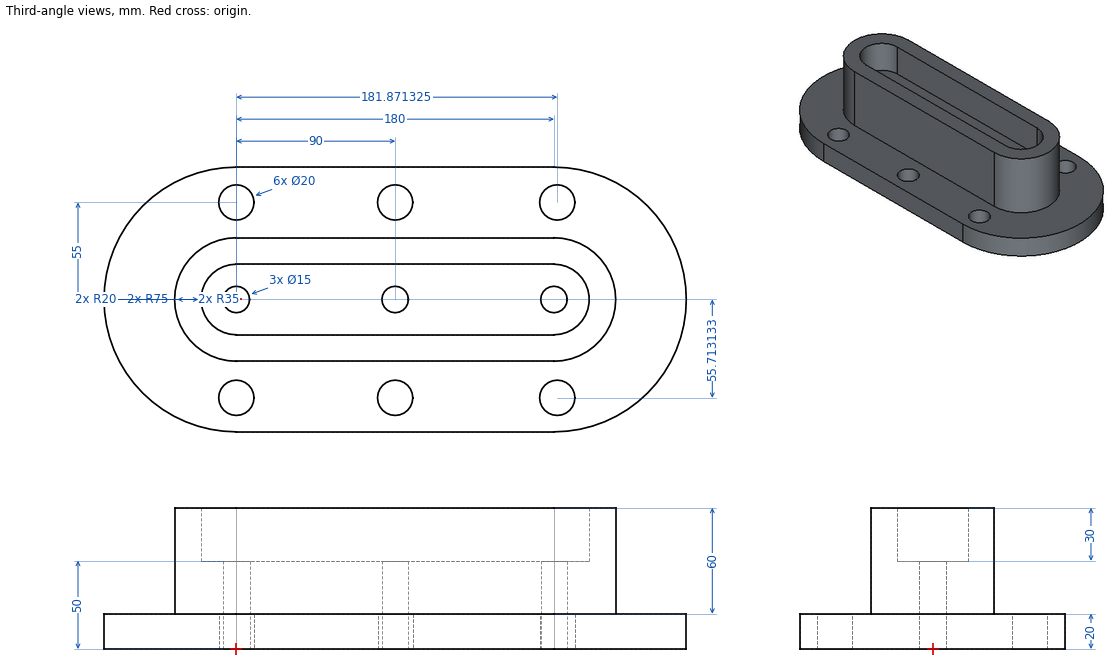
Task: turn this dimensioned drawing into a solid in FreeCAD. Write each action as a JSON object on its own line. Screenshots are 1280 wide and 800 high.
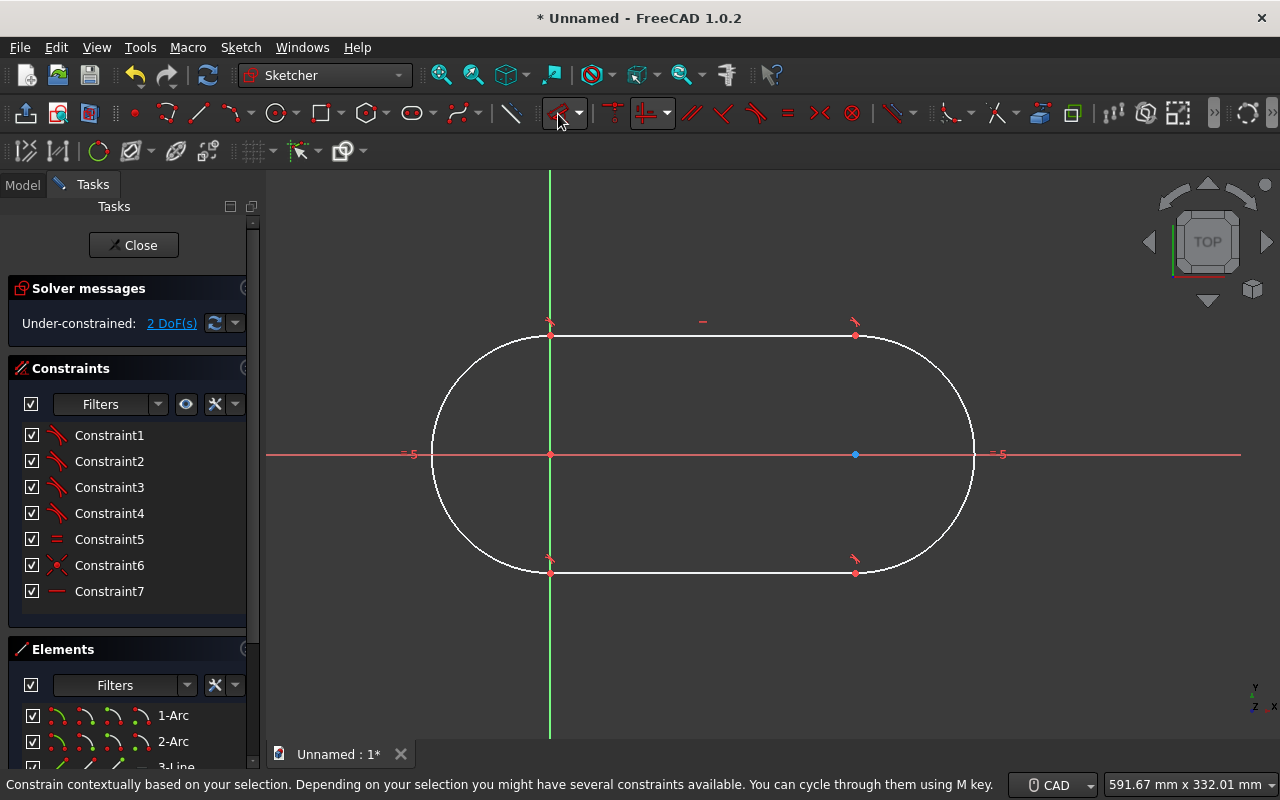
{"action": "left_click", "coordinate": [454, 385]}
{"action": "left_click", "coordinate": [428, 366]}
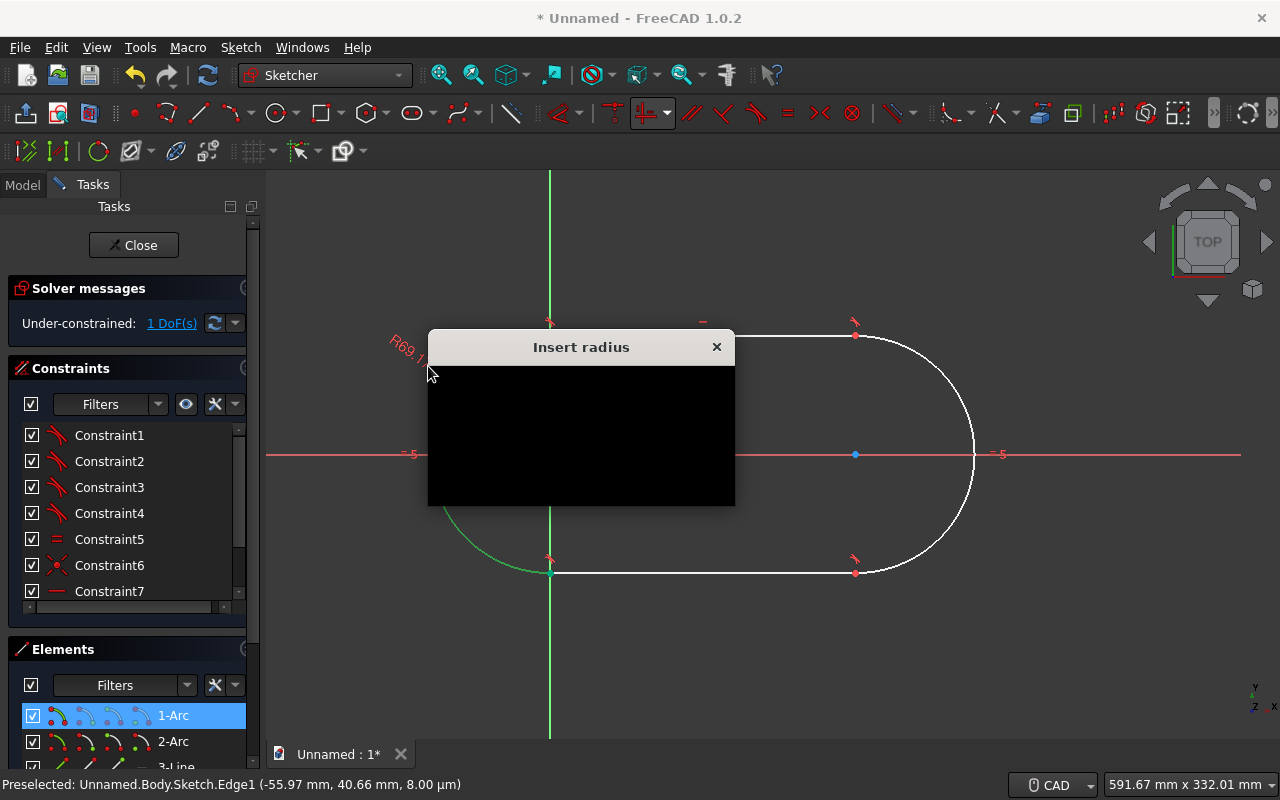
{"action": "type", "text": "75"}
{"action": "key", "text": "Return"}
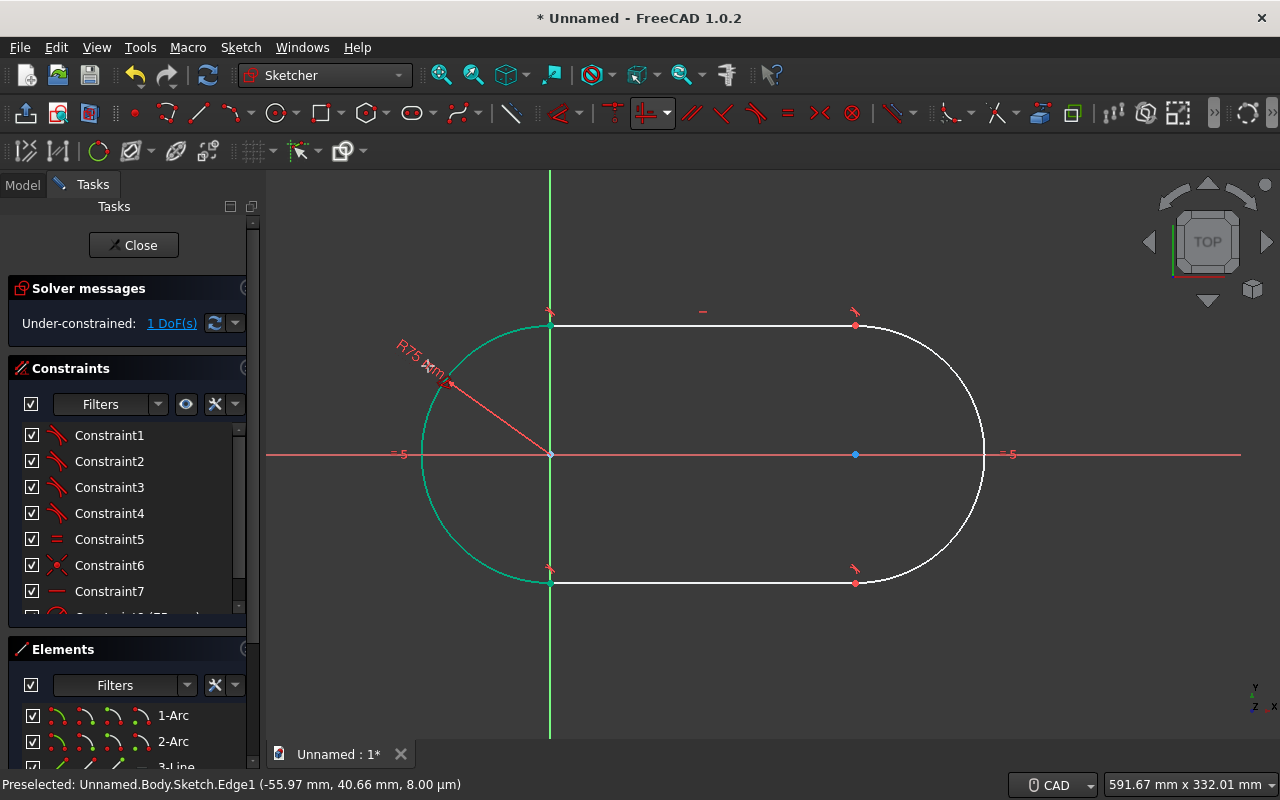
{"action": "left_click", "coordinate": [642, 326]}
{"action": "left_click", "coordinate": [703, 292]}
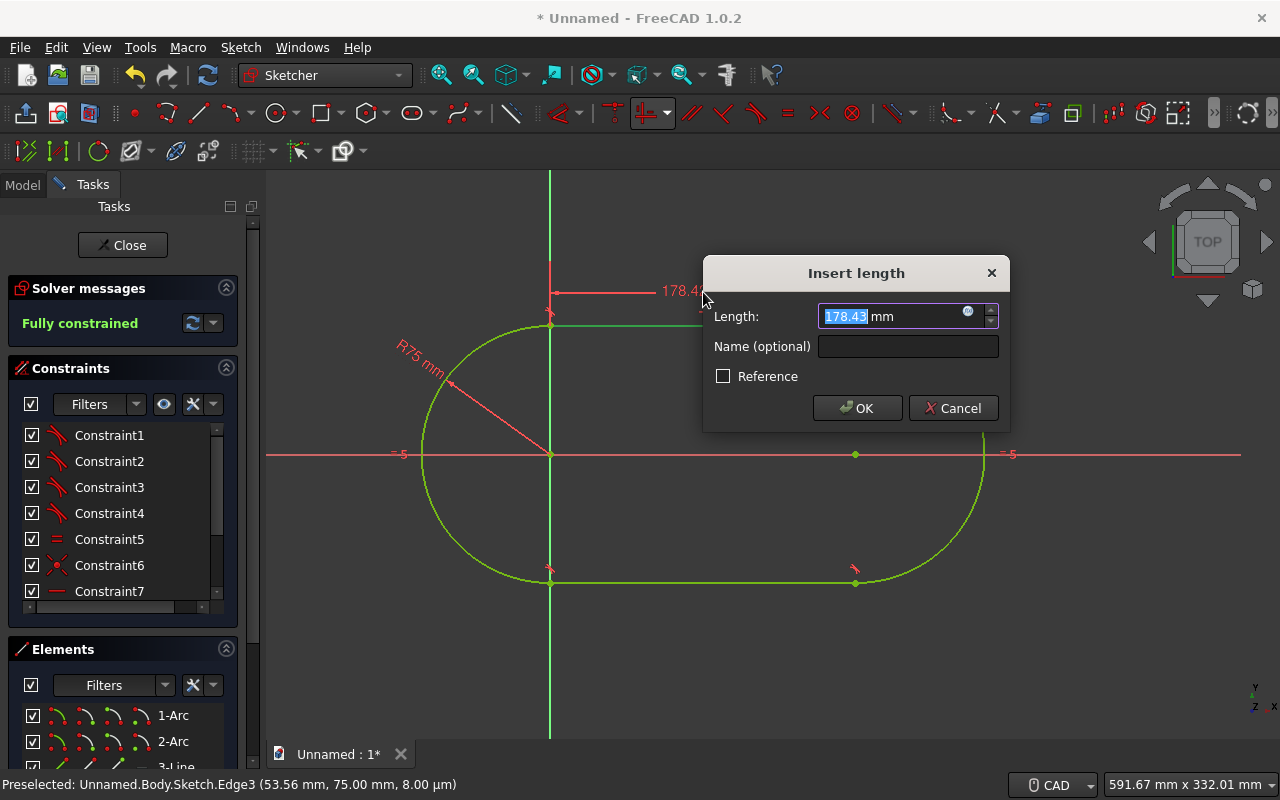
{"action": "type", "text": "180"}
{"action": "key", "text": "Return"}
{"action": "key", "text": "Escape"}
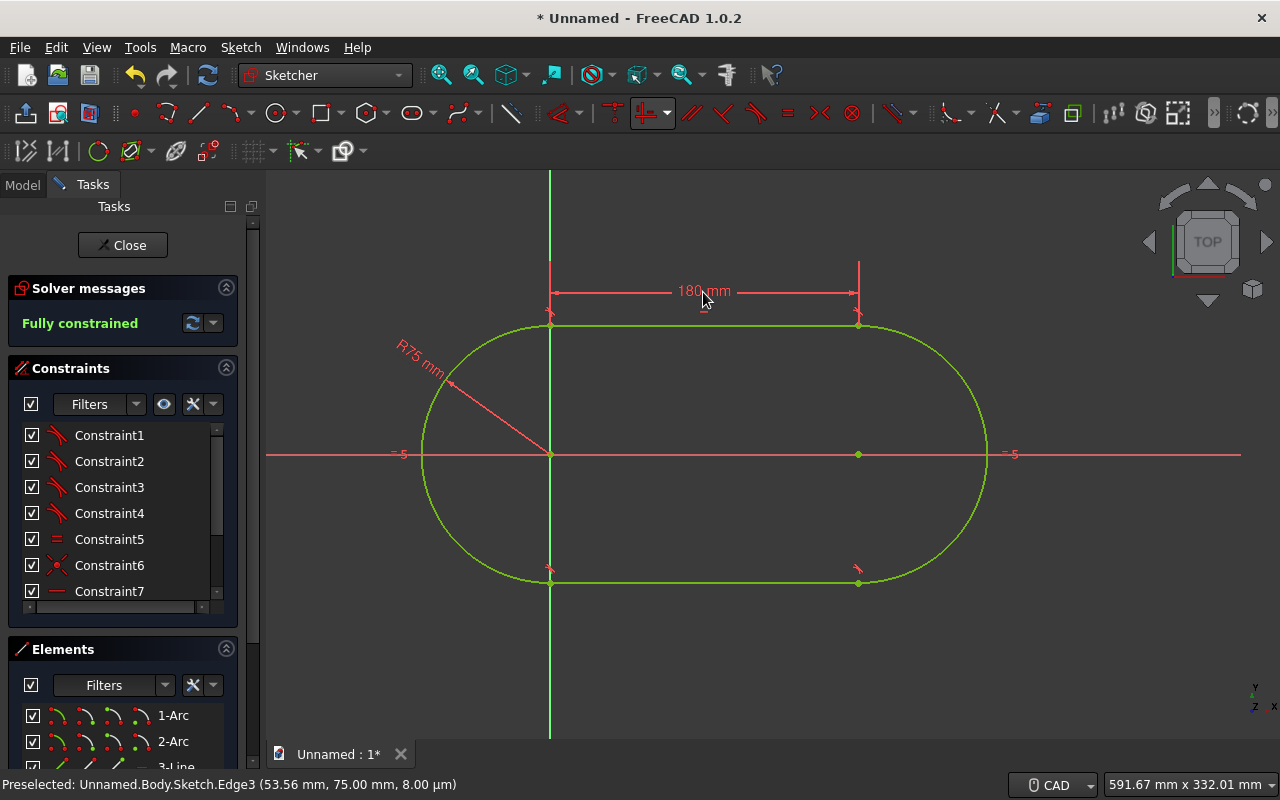
{"action": "left_click", "coordinate": [123, 245]}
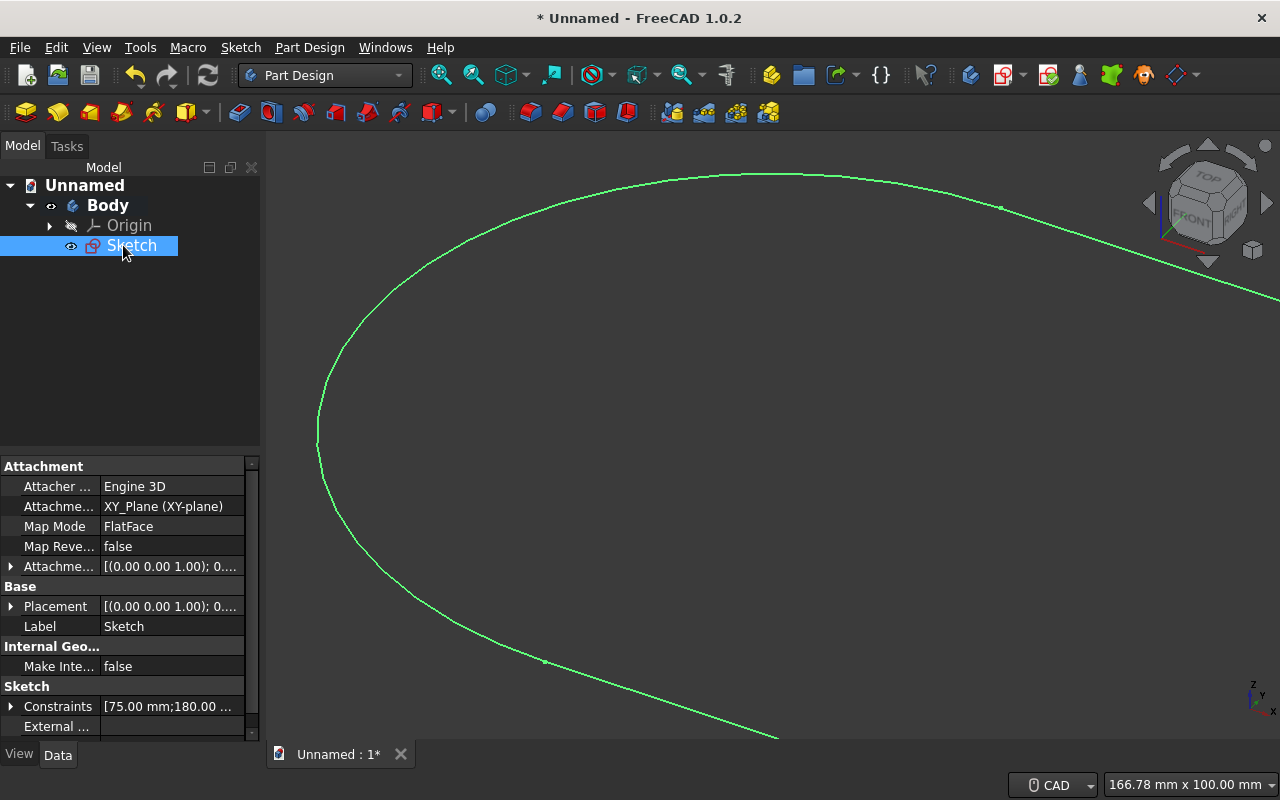
{"action": "left_click", "coordinate": [26, 112]}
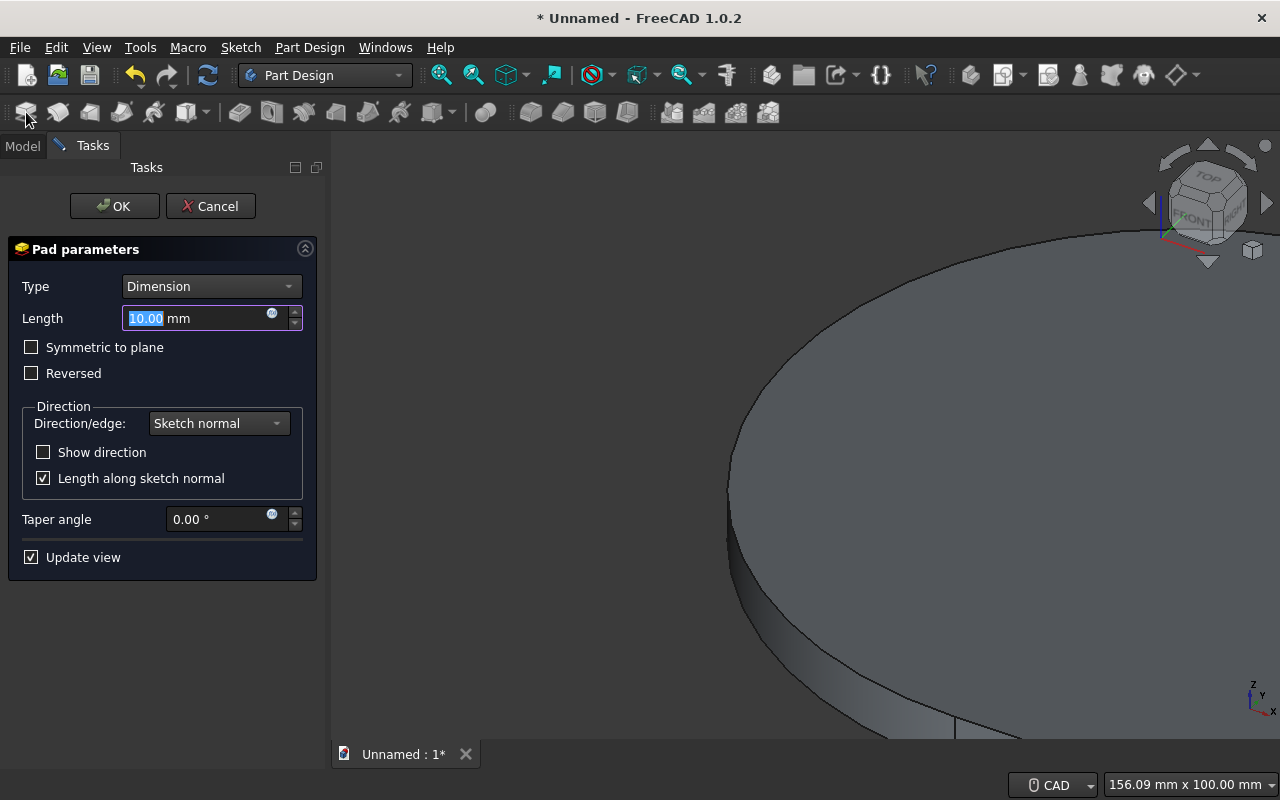
{"action": "type", "text": "20"}
{"action": "key", "text": "Tab"}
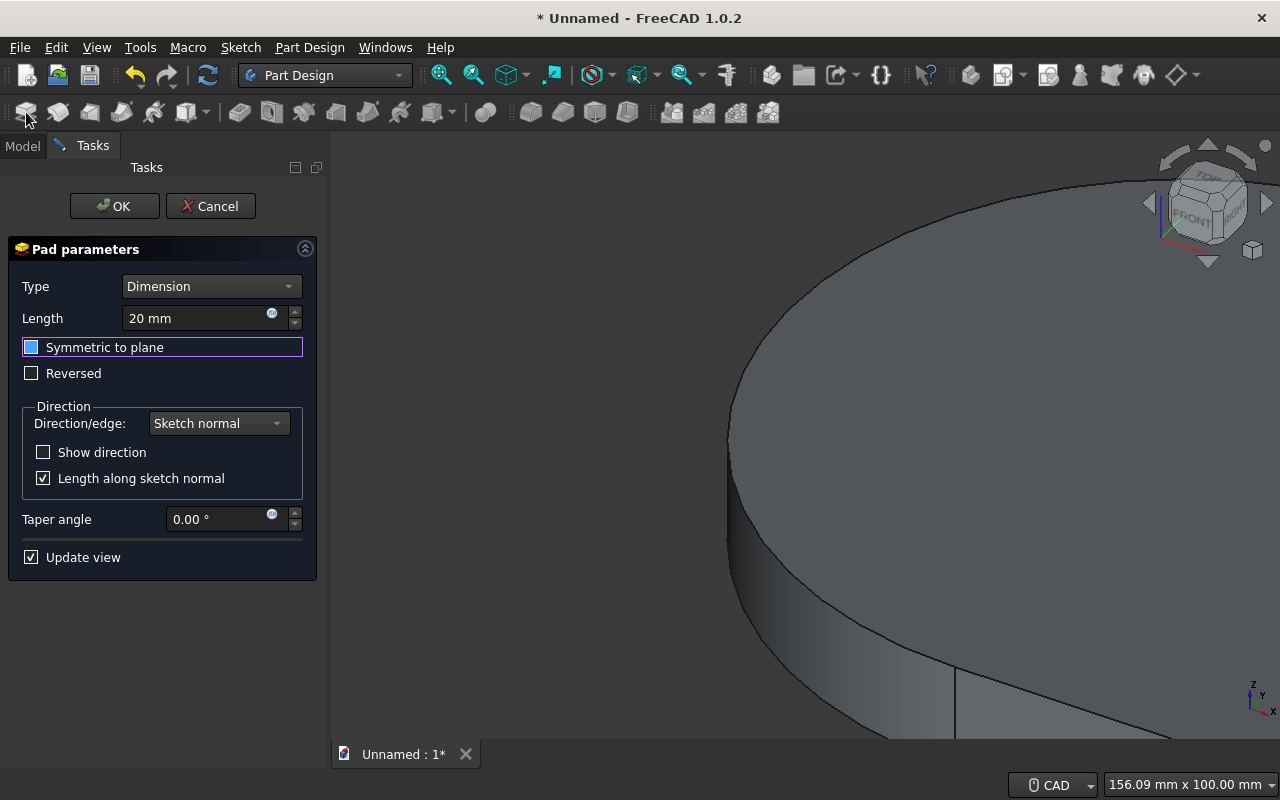
{"action": "left_click", "coordinate": [115, 206]}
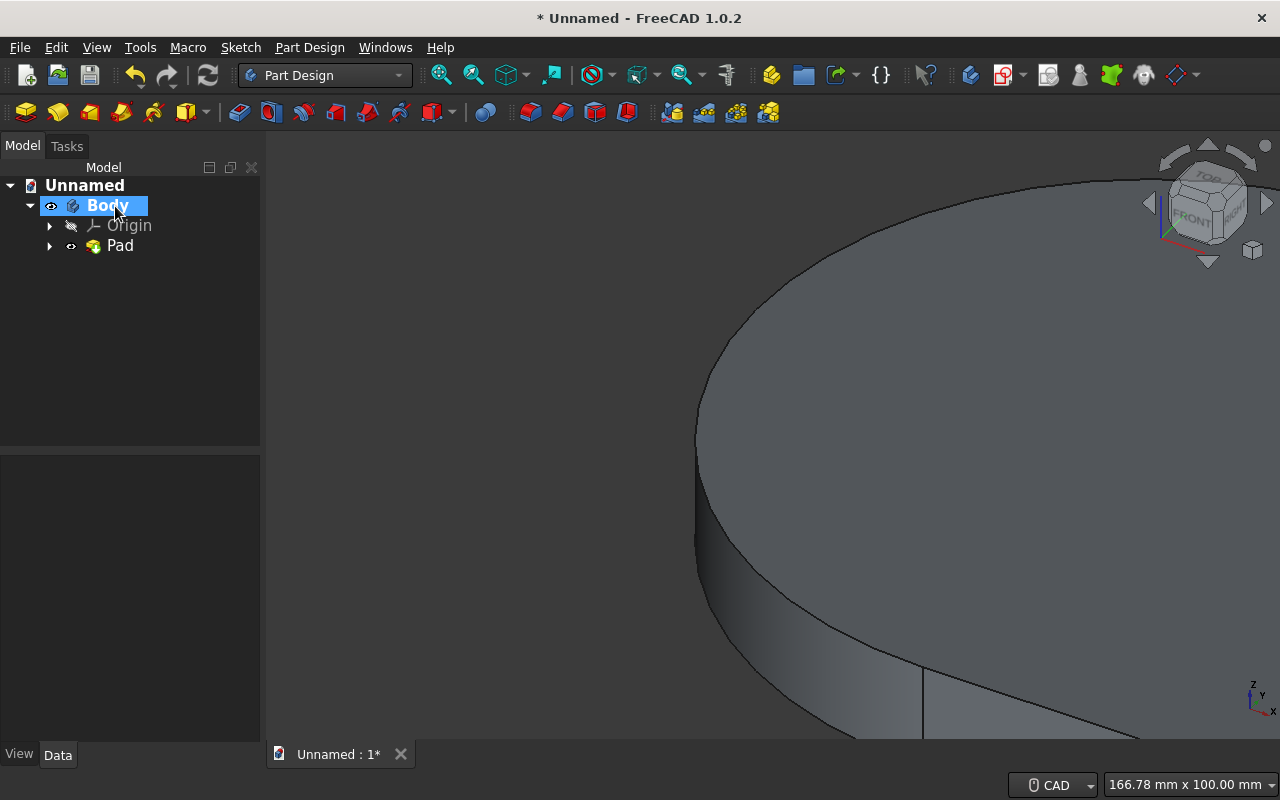
{"action": "left_click", "coordinate": [442, 76]}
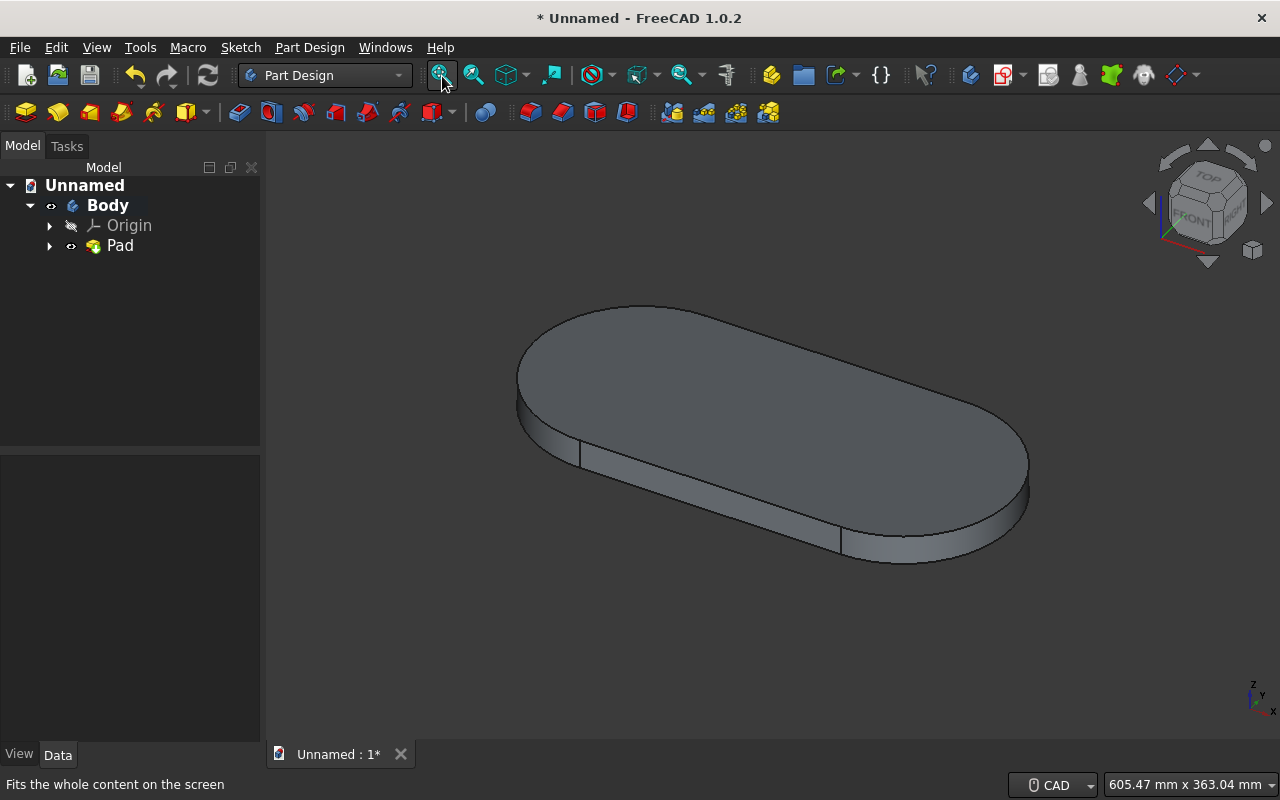
{"action": "left_click", "coordinate": [841, 443]}